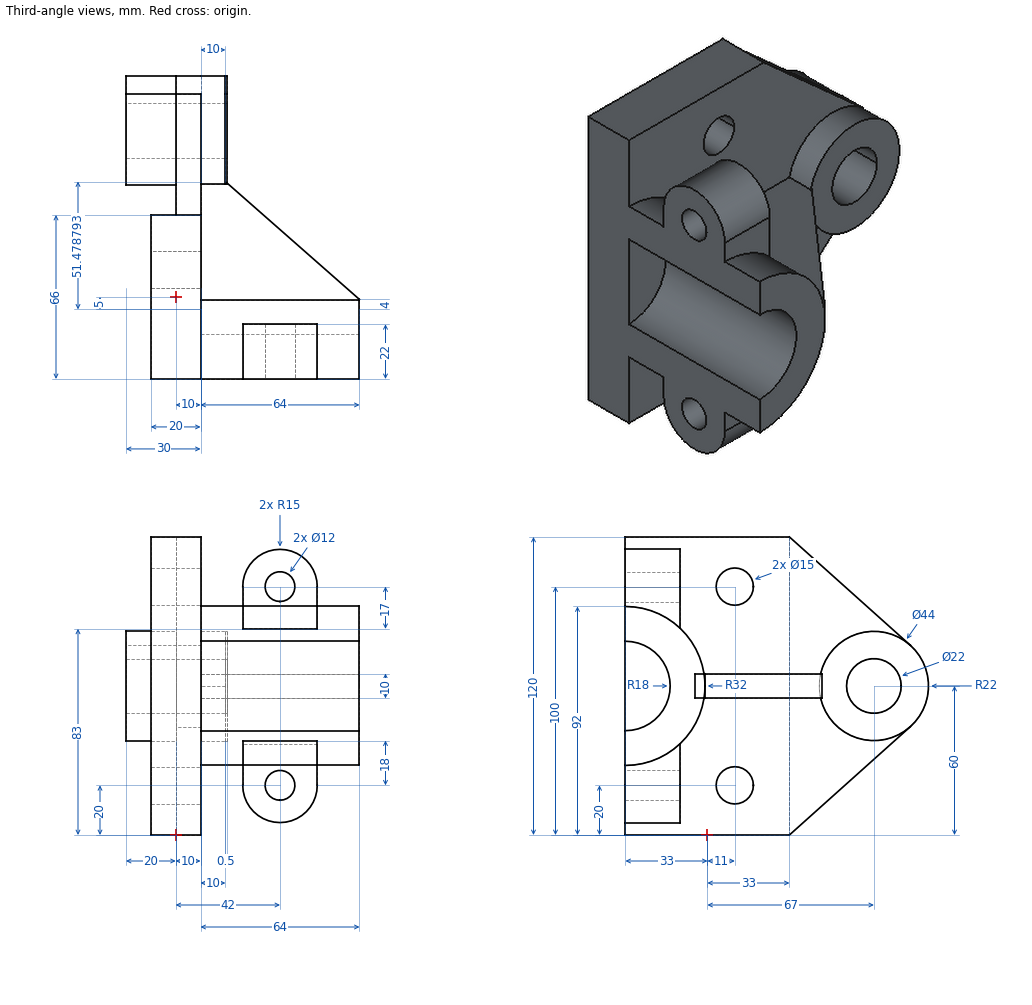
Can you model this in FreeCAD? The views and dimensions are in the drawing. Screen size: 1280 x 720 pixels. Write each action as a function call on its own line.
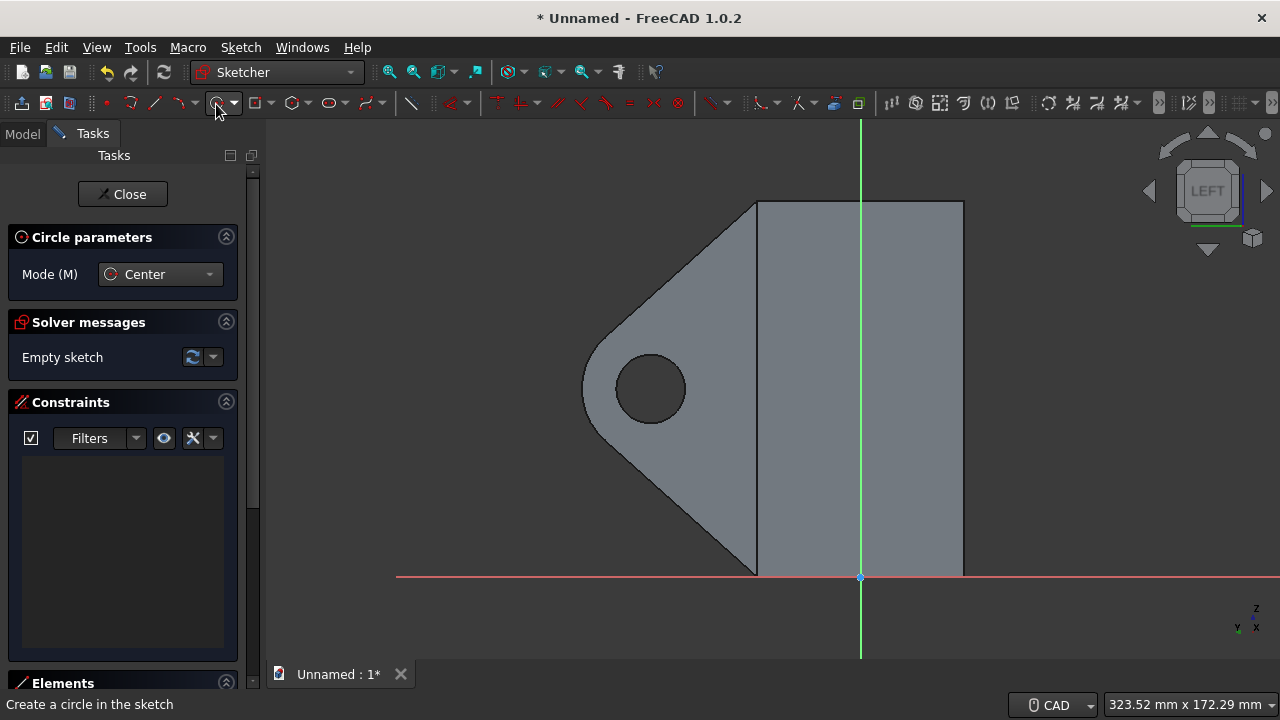
click(651, 389)
click(700, 340)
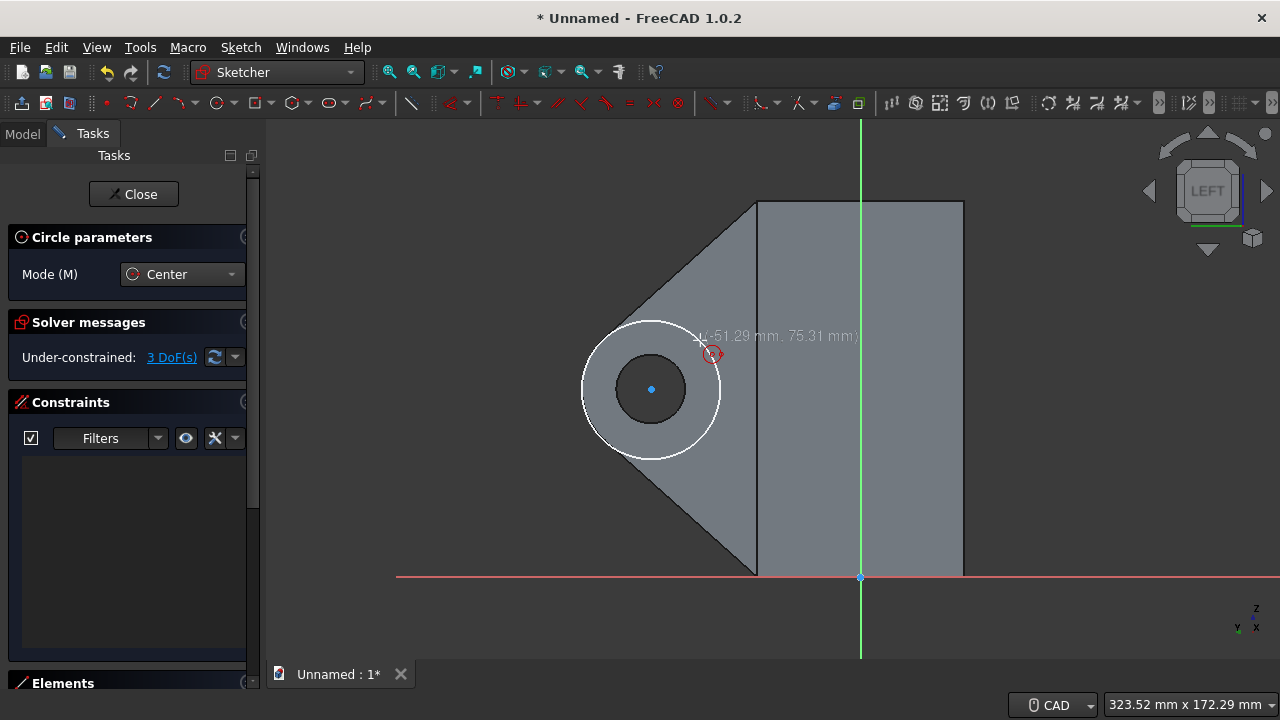
click(651, 390)
click(675, 365)
key(Escape)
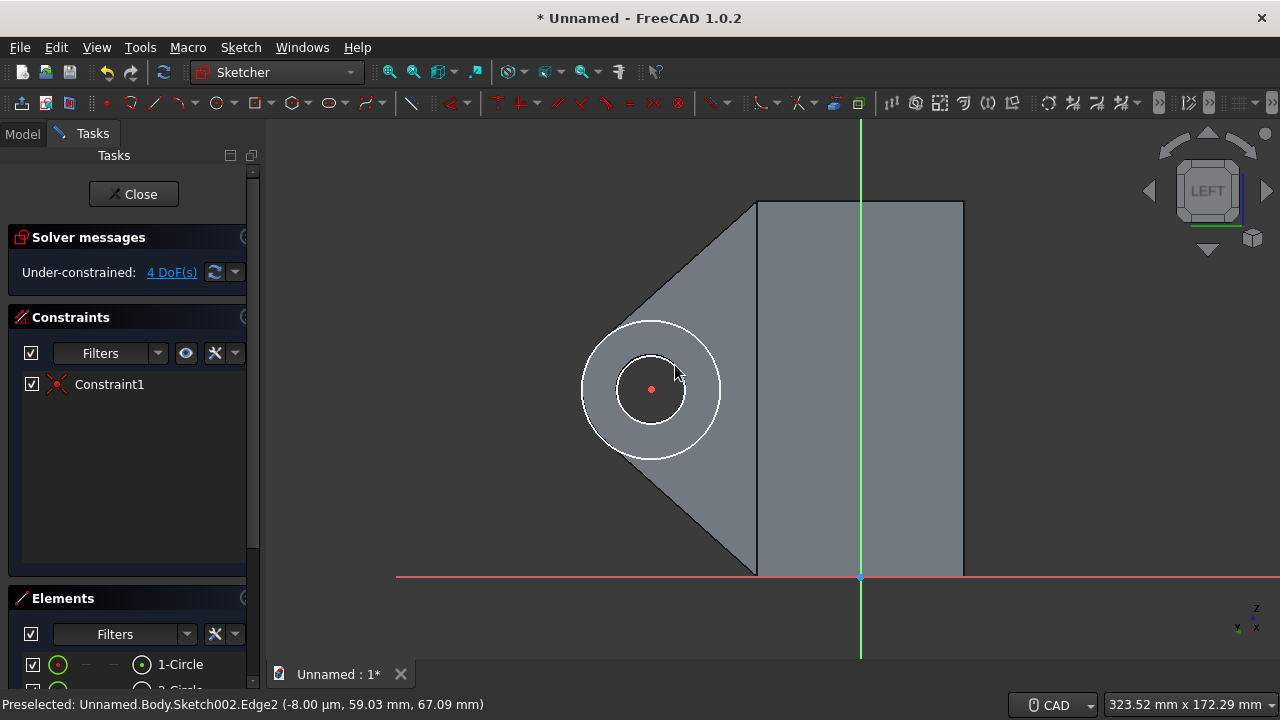
click(450, 104)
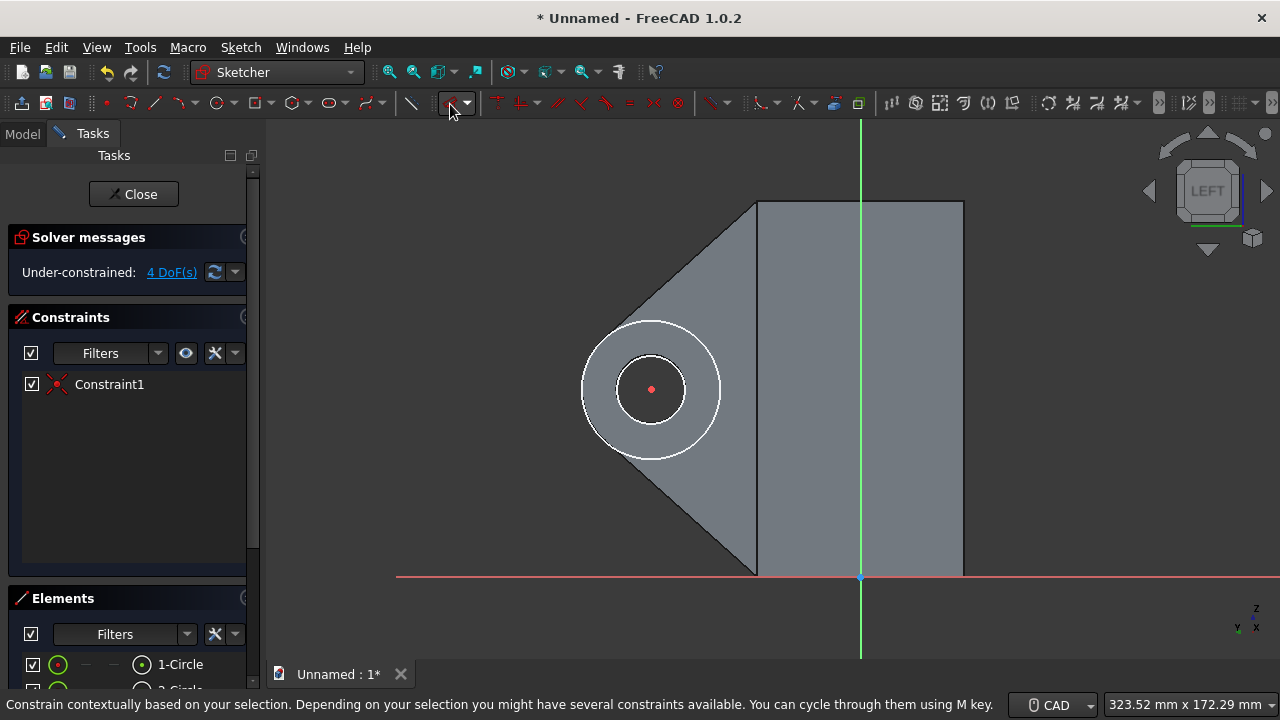
click(700, 341)
click(723, 318)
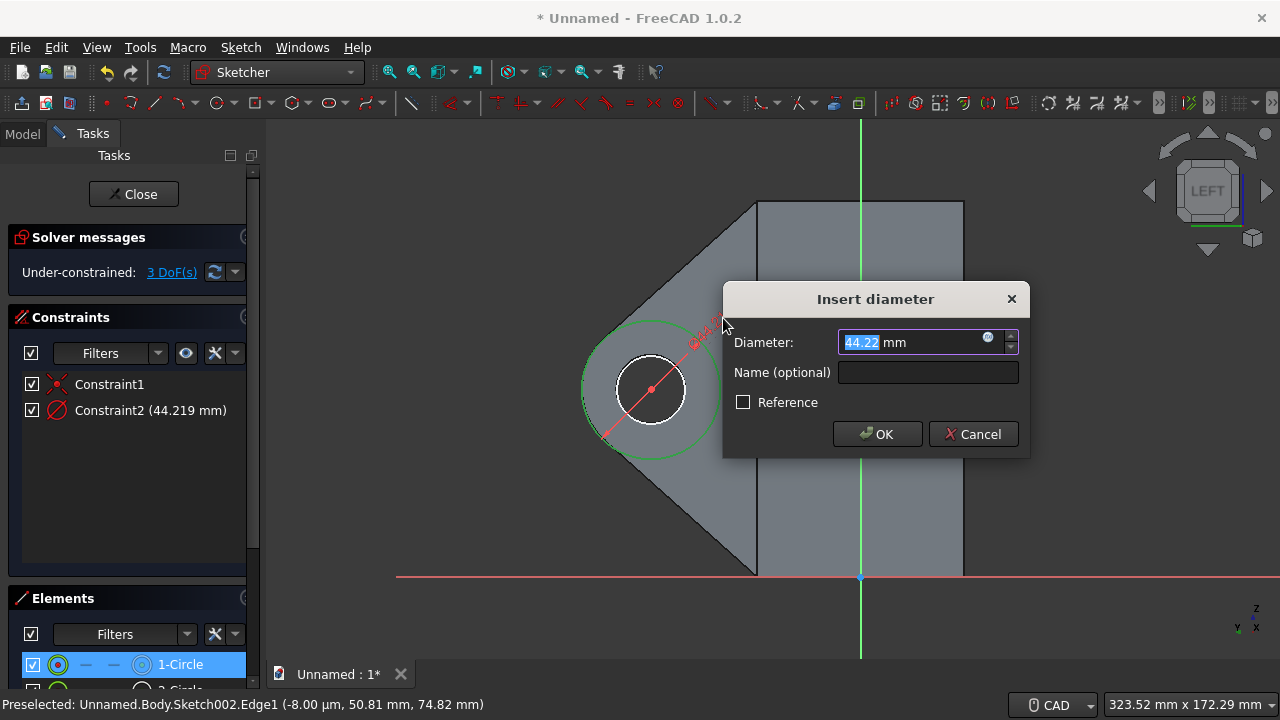
text(44)
key(Return)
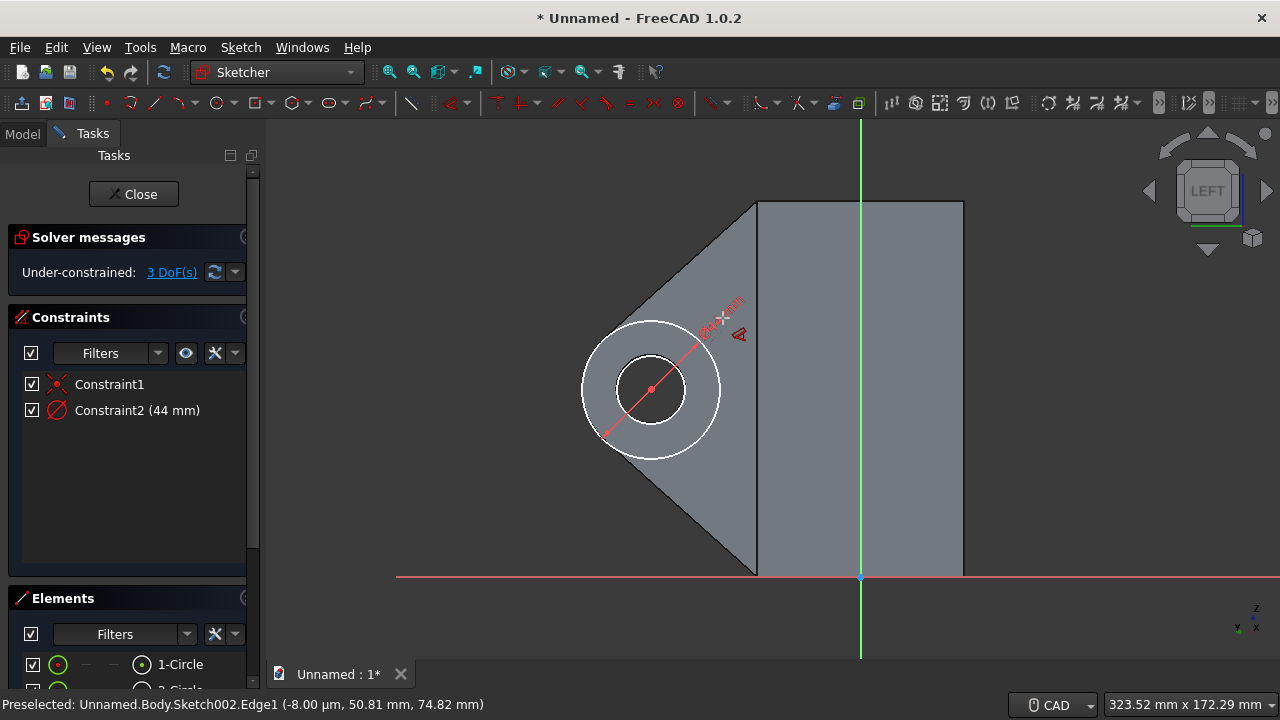
click(675, 366)
click(736, 365)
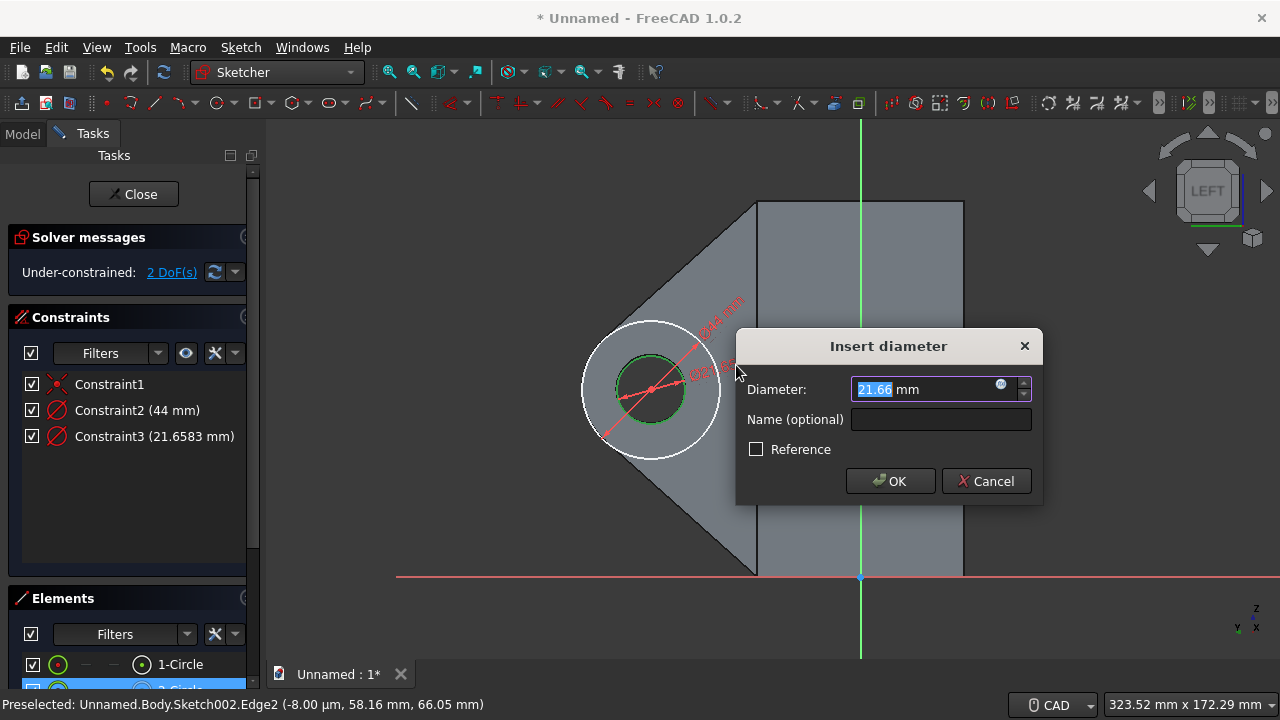
text(22)
key(Return)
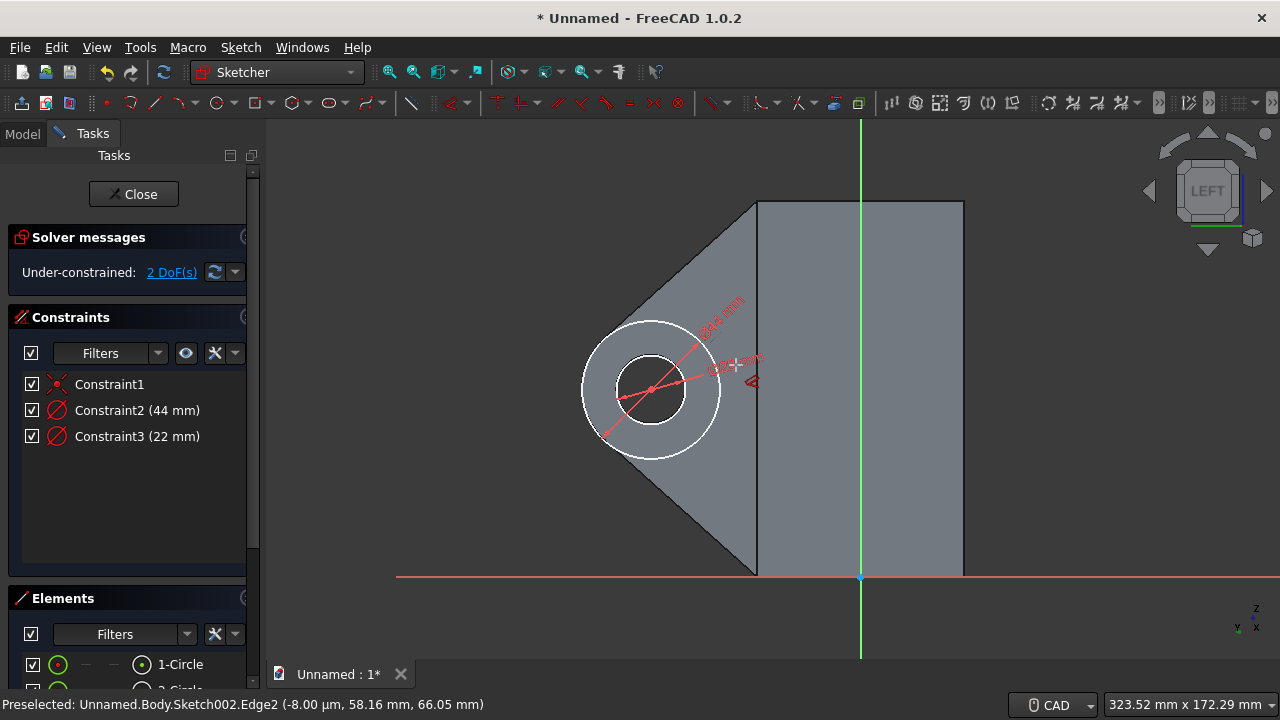
click(651, 390)
click(756, 611)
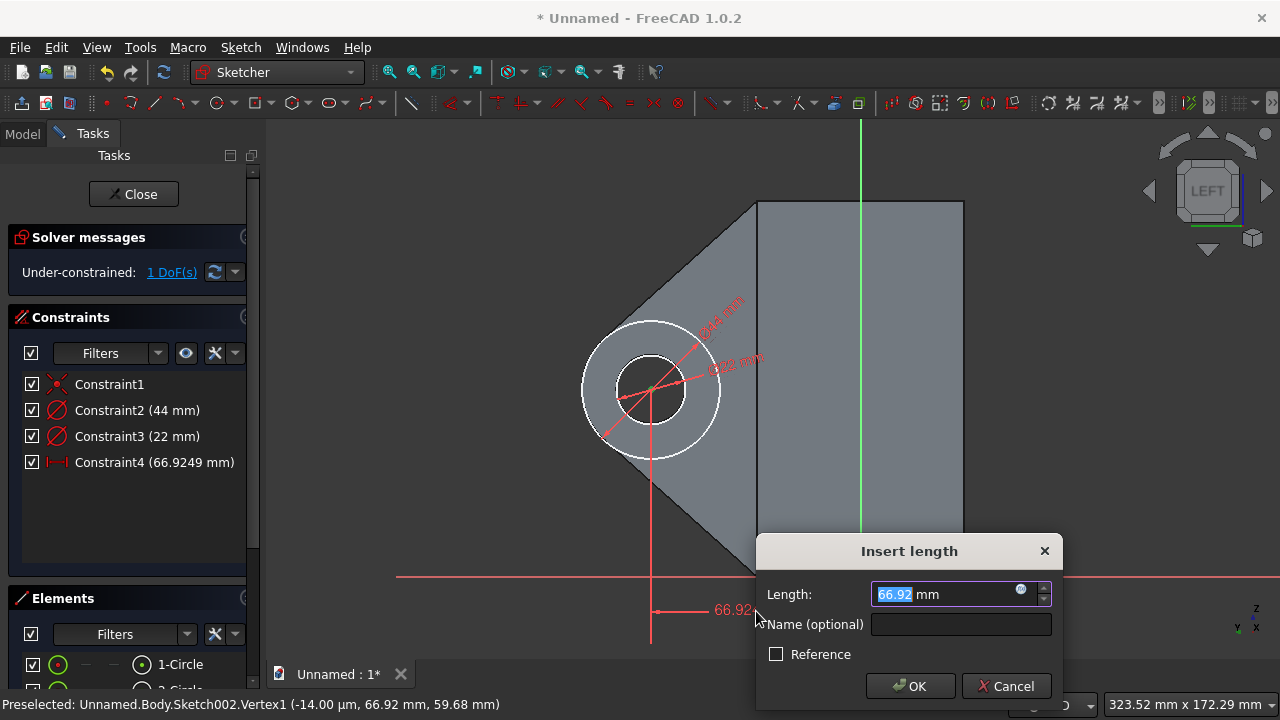
text(67)
key(Return)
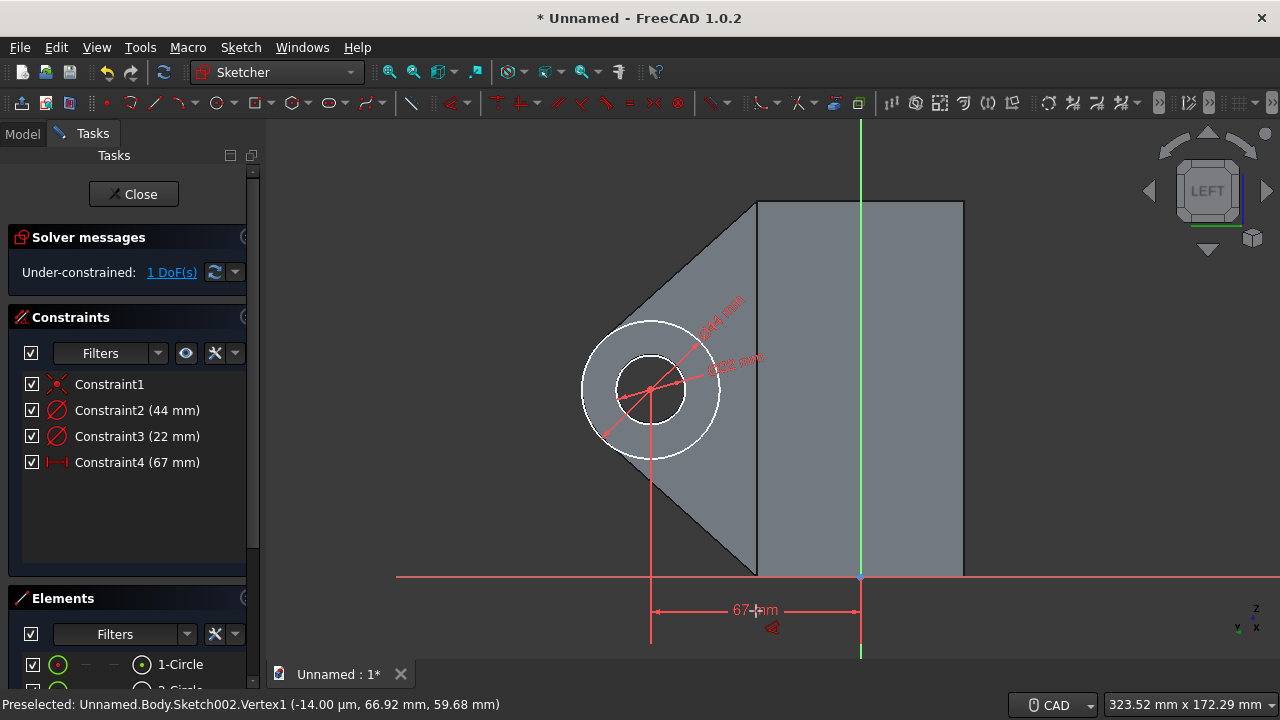
click(651, 390)
click(895, 484)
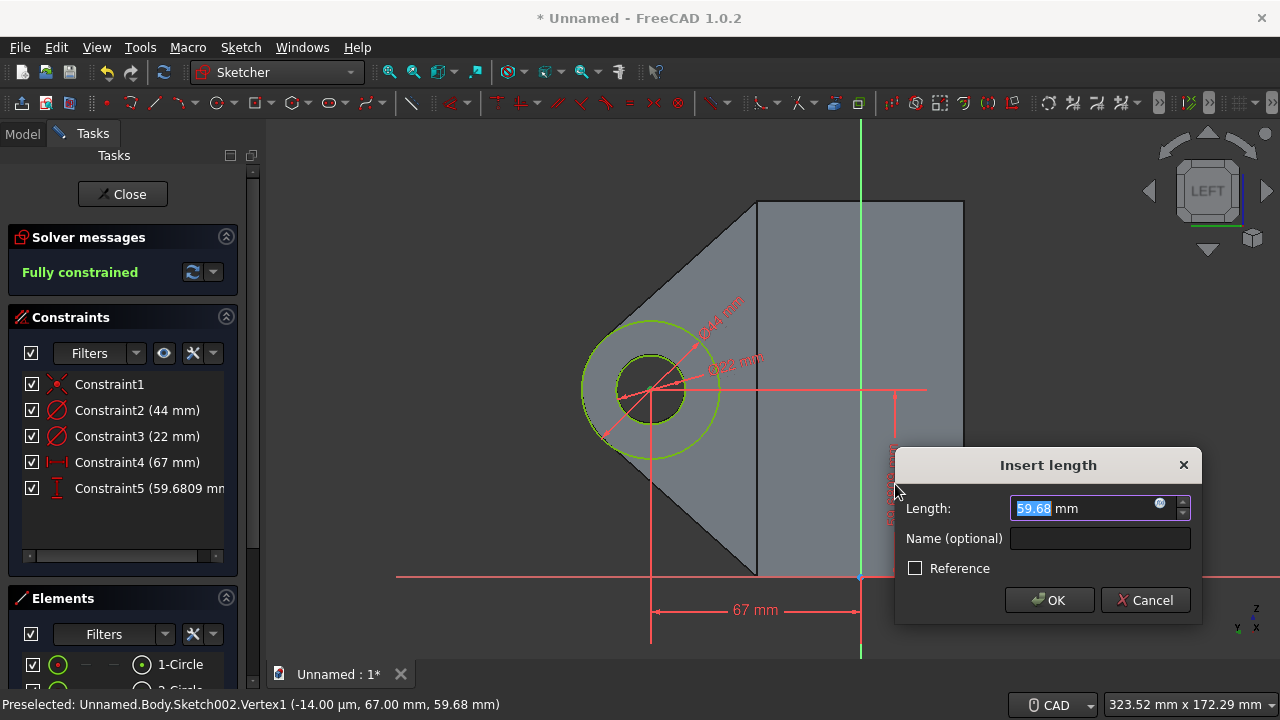
text(60)
key(Return)
key(Escape)